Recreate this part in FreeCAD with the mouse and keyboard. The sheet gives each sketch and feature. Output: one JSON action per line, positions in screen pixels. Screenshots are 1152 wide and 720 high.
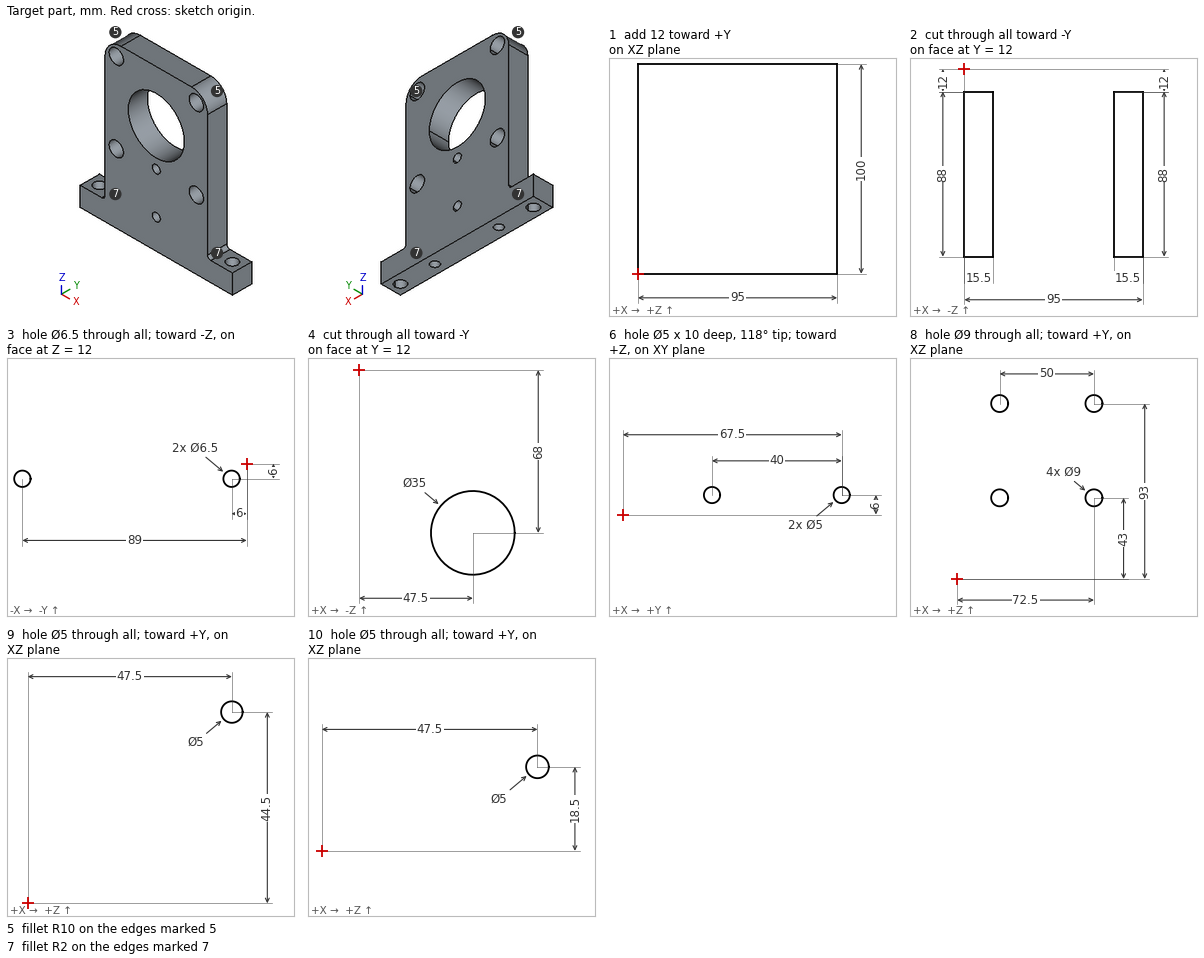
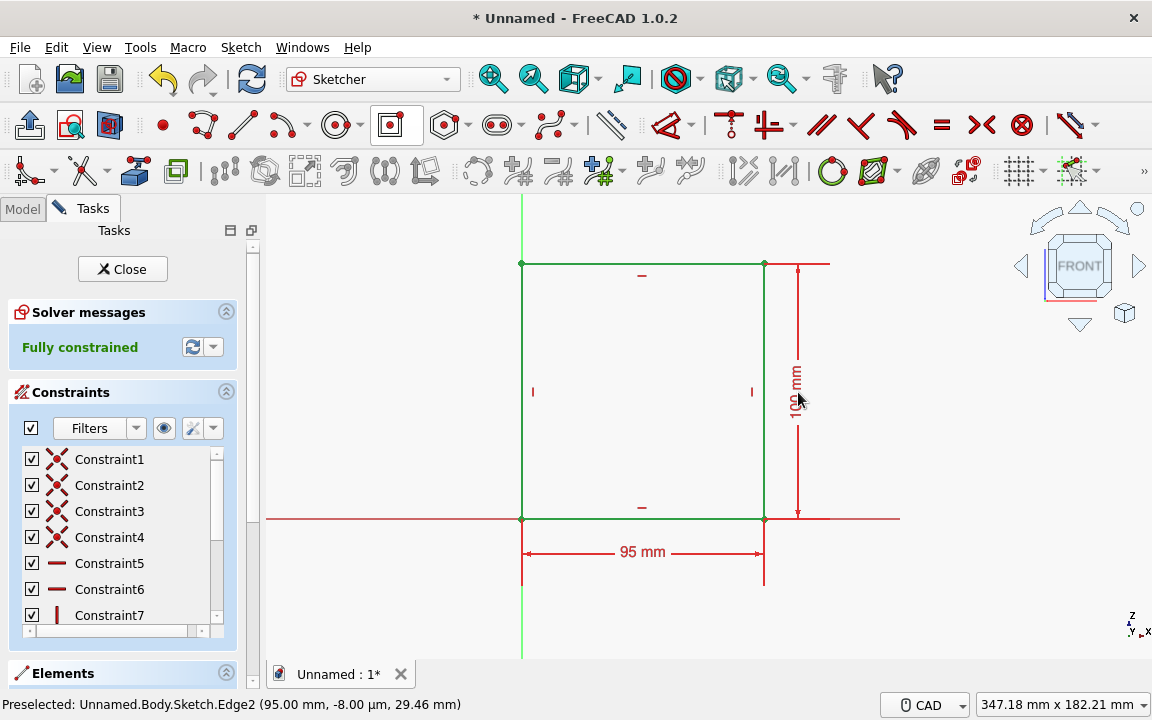
{"action": "left_click", "coordinate": [123, 269]}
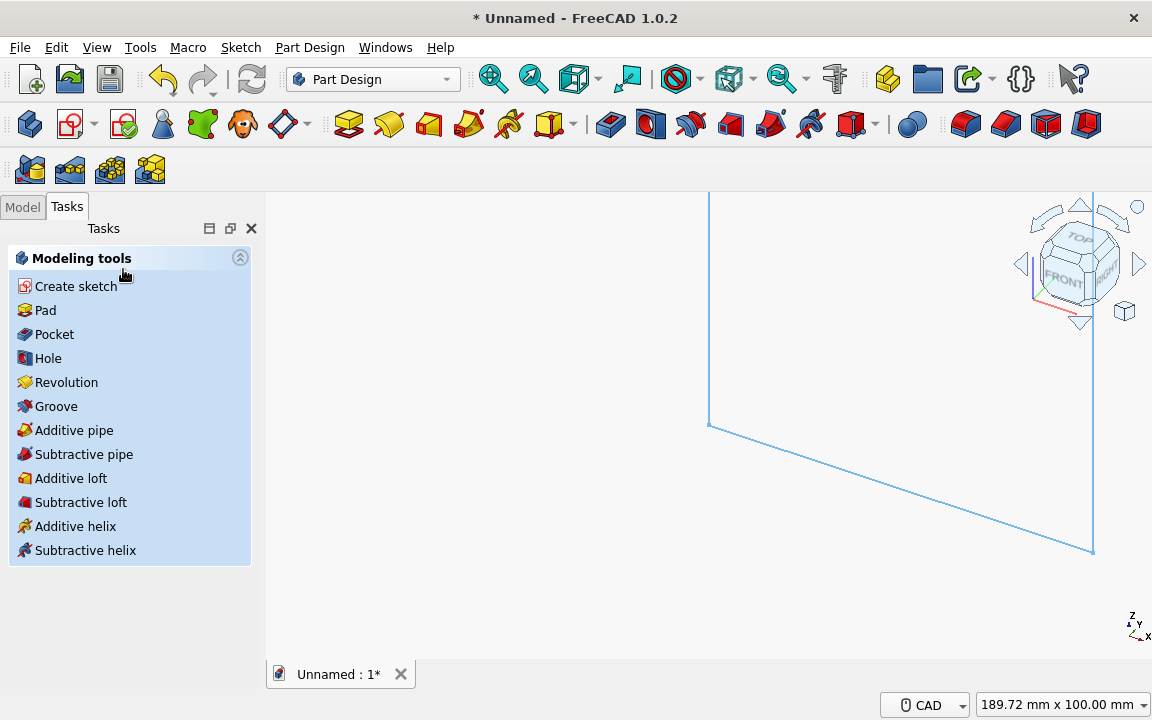
{"action": "left_click", "coordinate": [350, 124]}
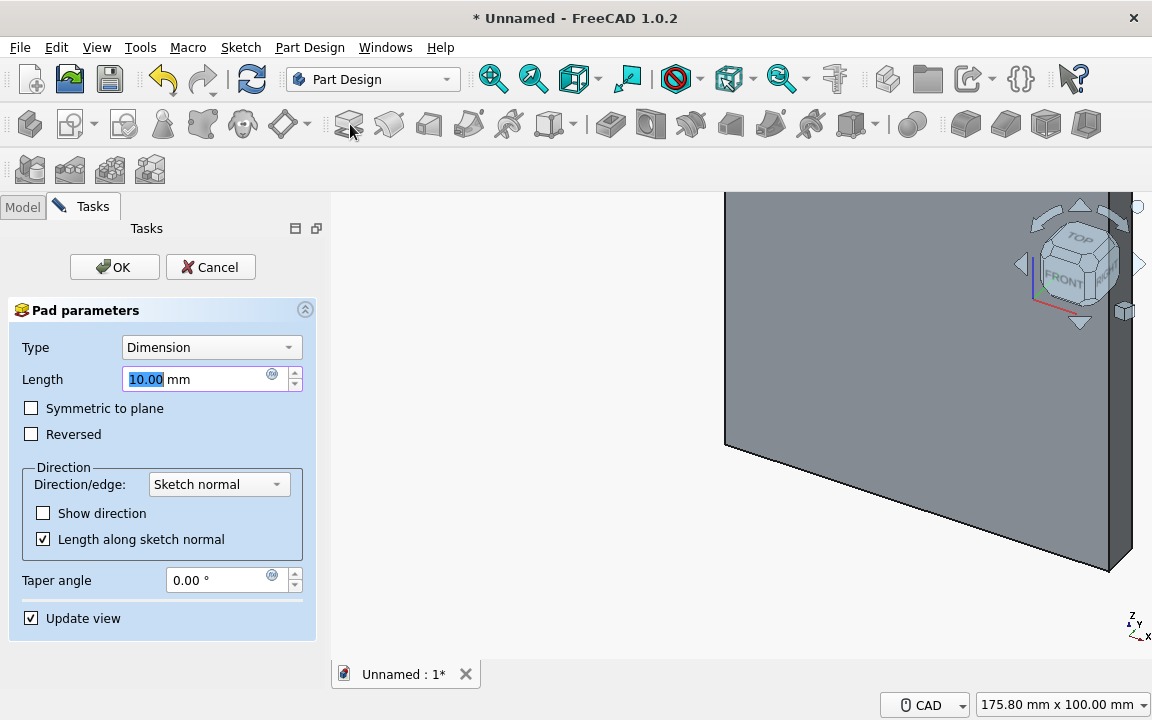
{"action": "type", "text": "12"}
{"action": "key", "text": "Tab"}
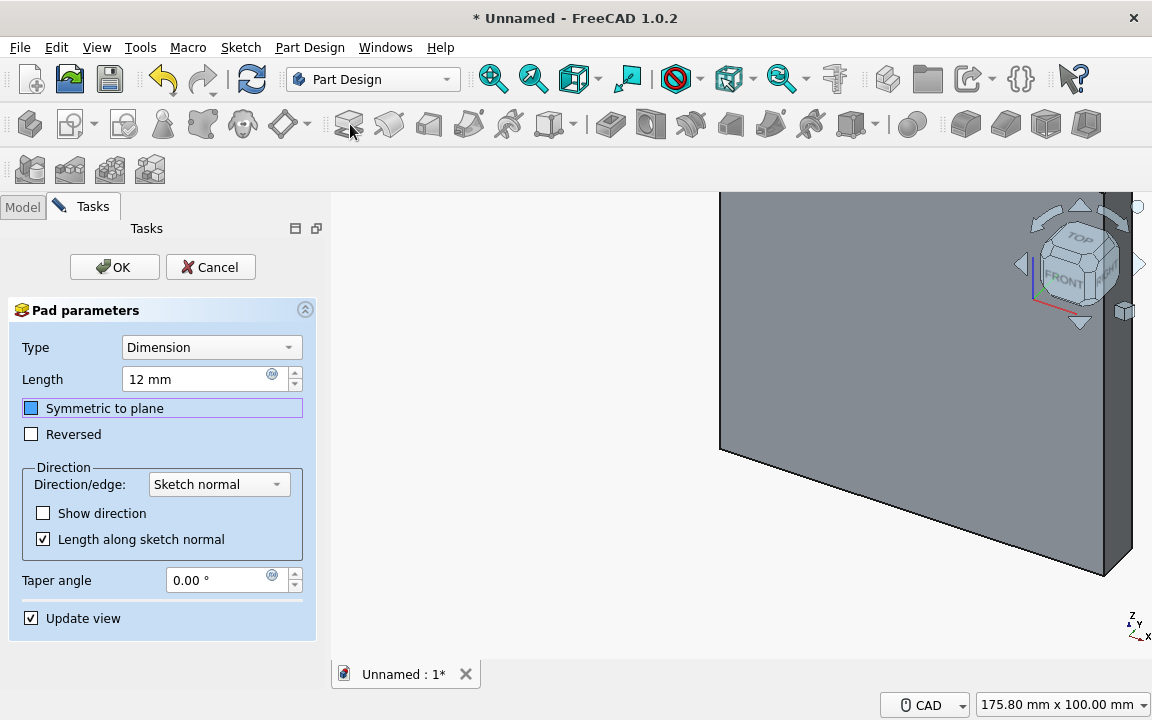
{"action": "left_click", "coordinate": [30, 434]}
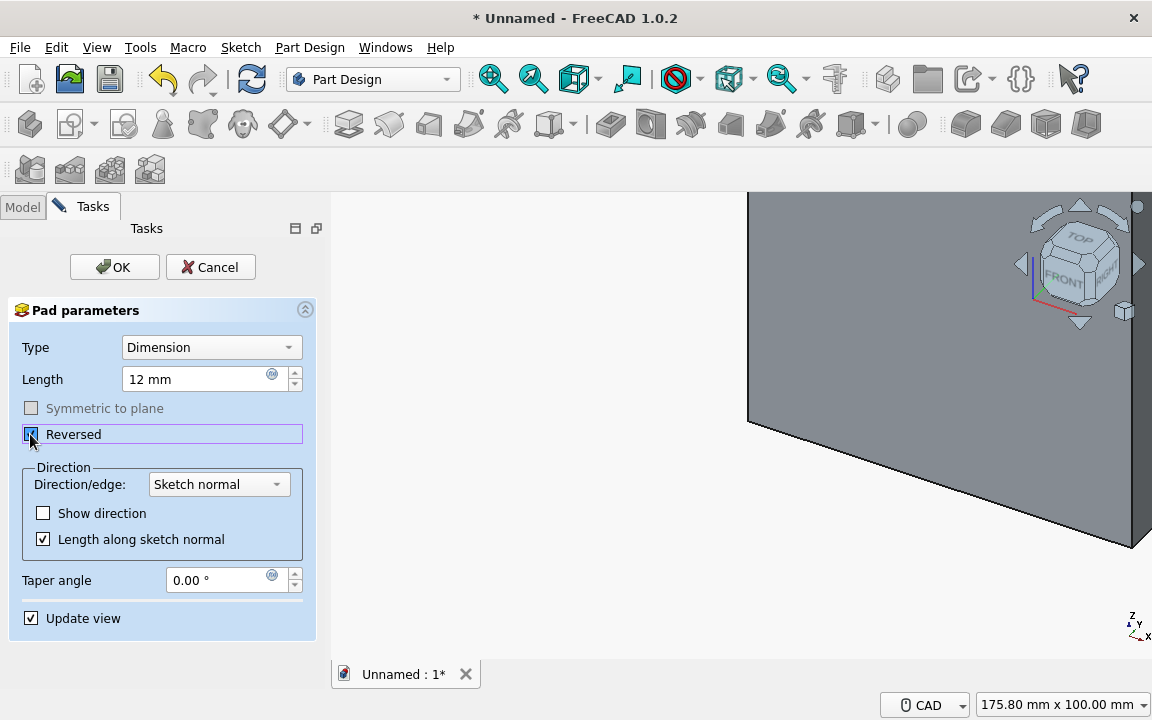
{"action": "left_click", "coordinate": [115, 267]}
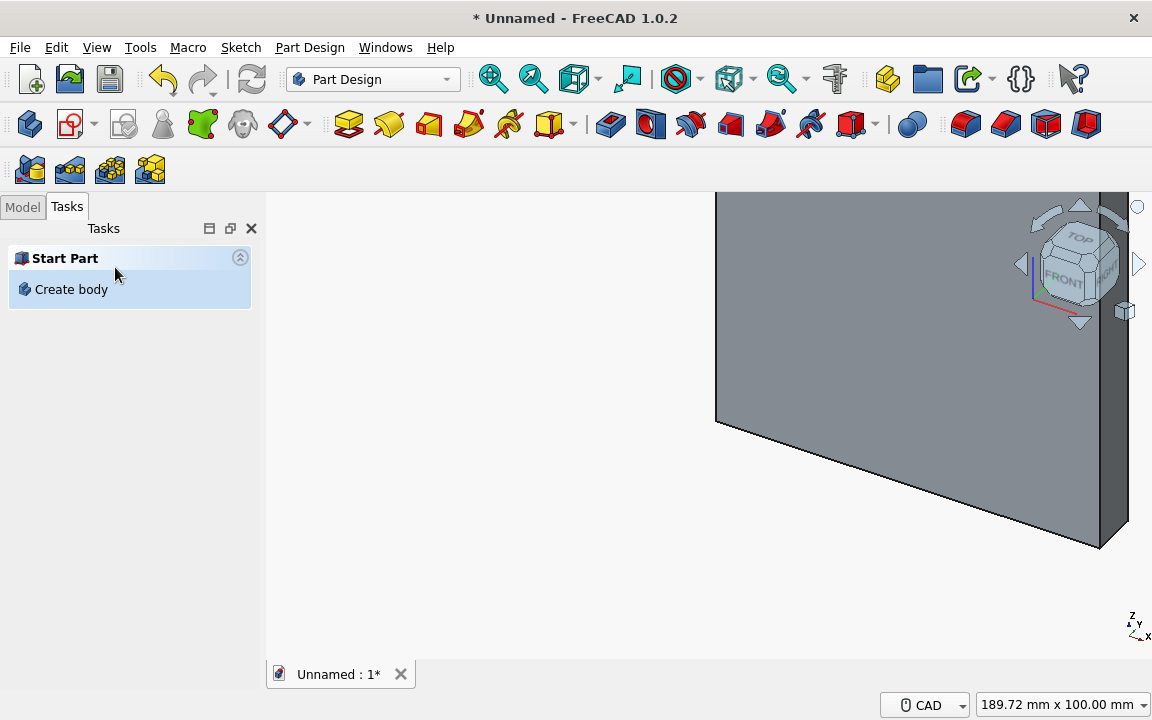
{"action": "left_click", "coordinate": [494, 80]}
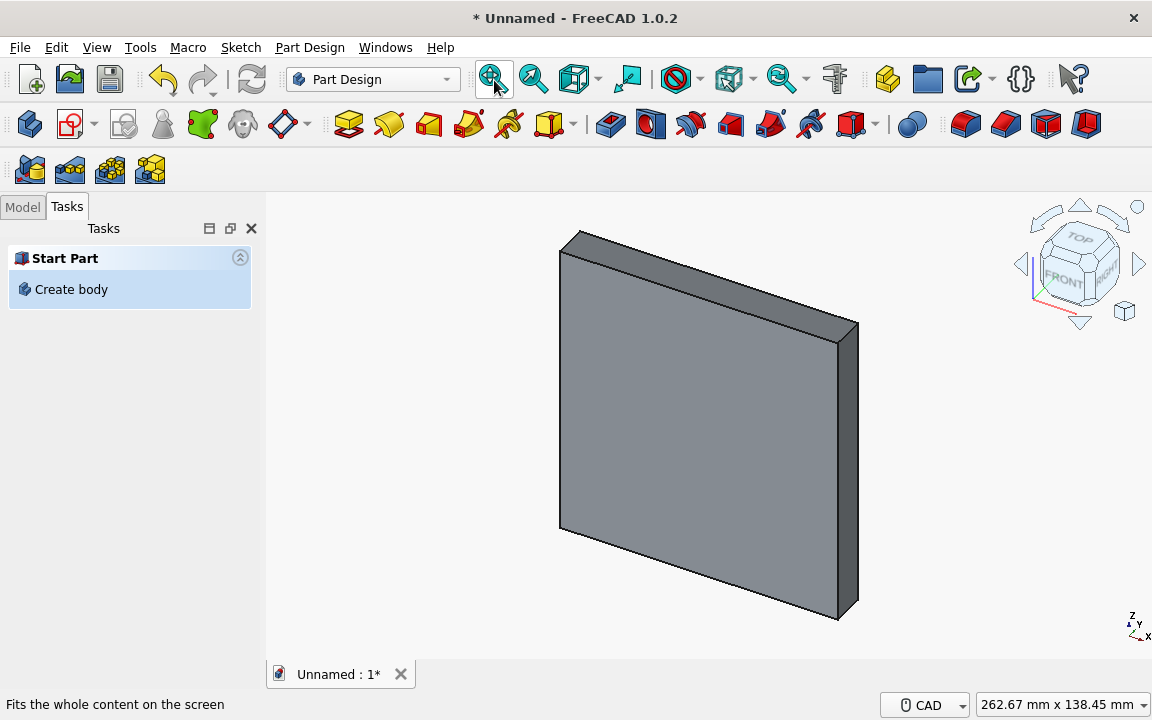
{"action": "key", "text": "4"}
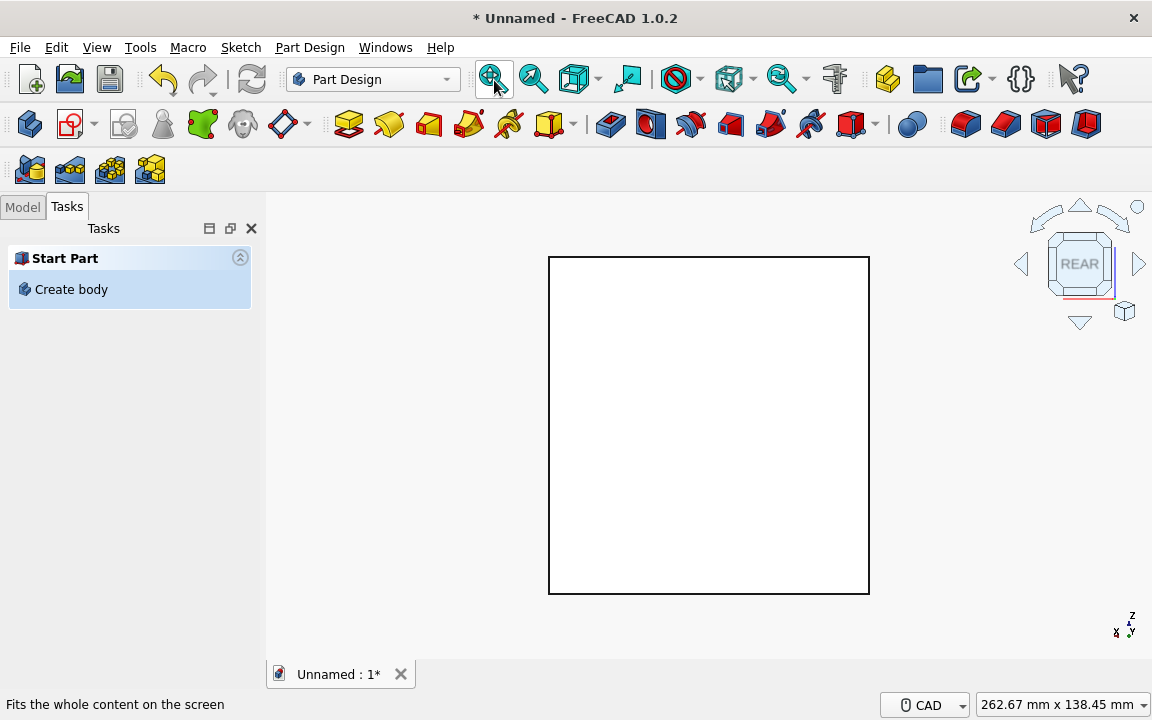
{"action": "left_click", "coordinate": [709, 425]}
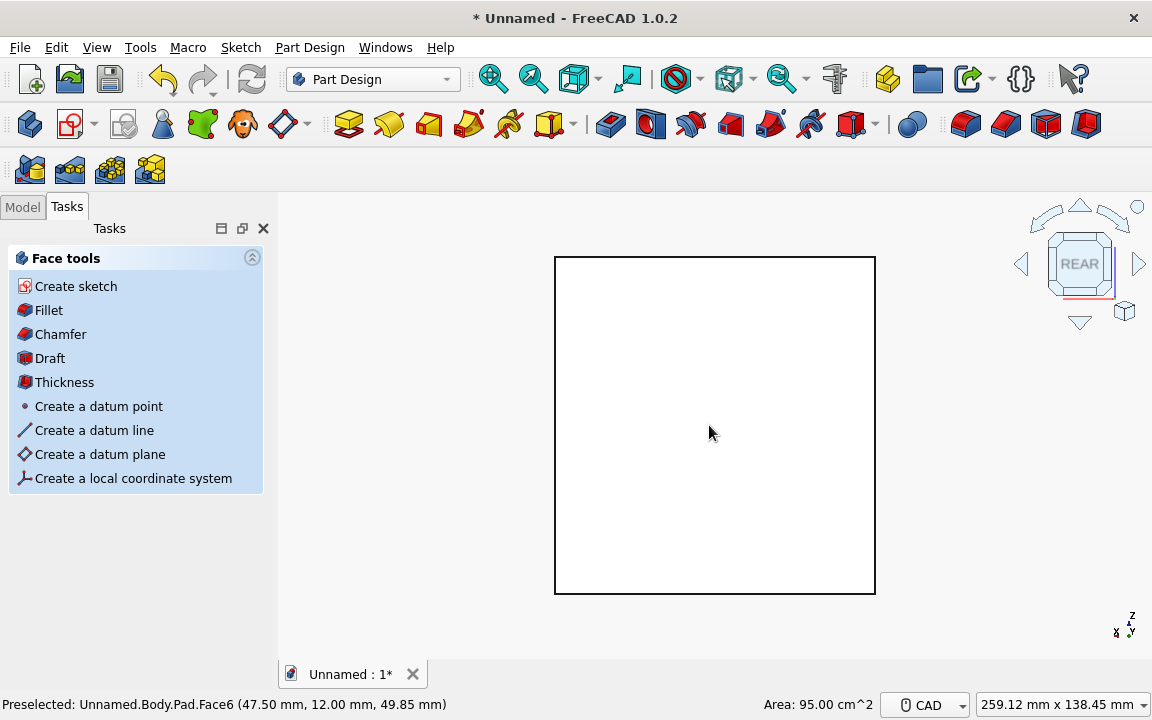
{"action": "left_click", "coordinate": [70, 124]}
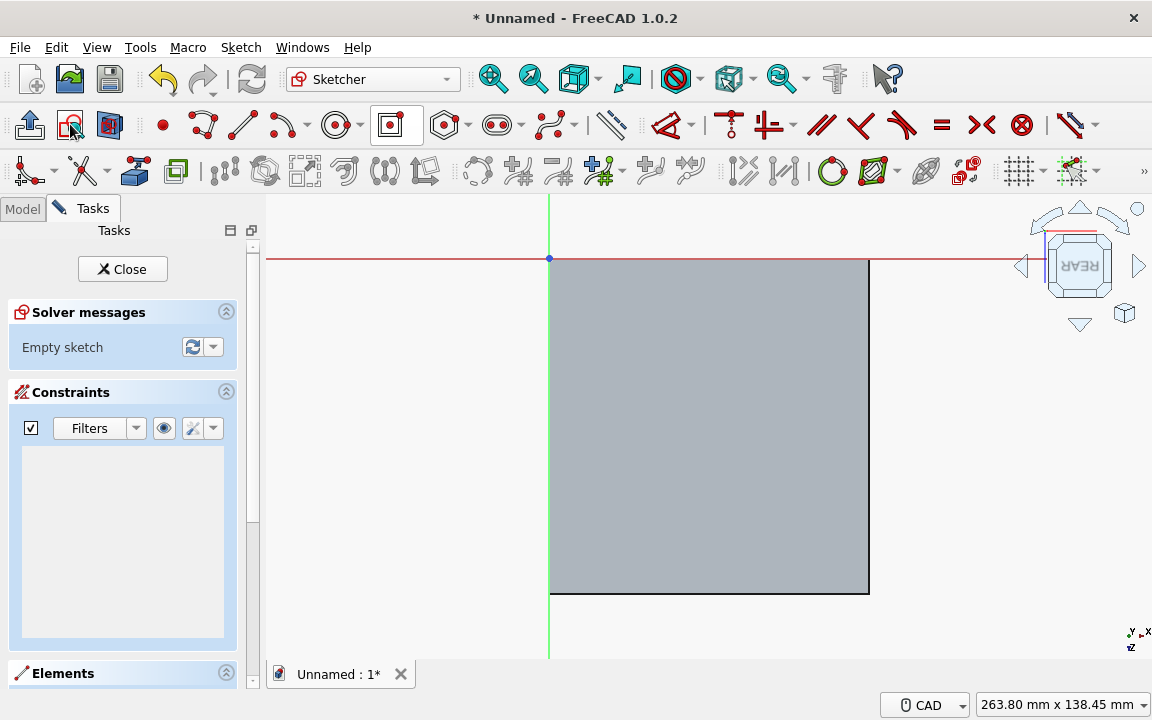
{"action": "key", "text": "g r"}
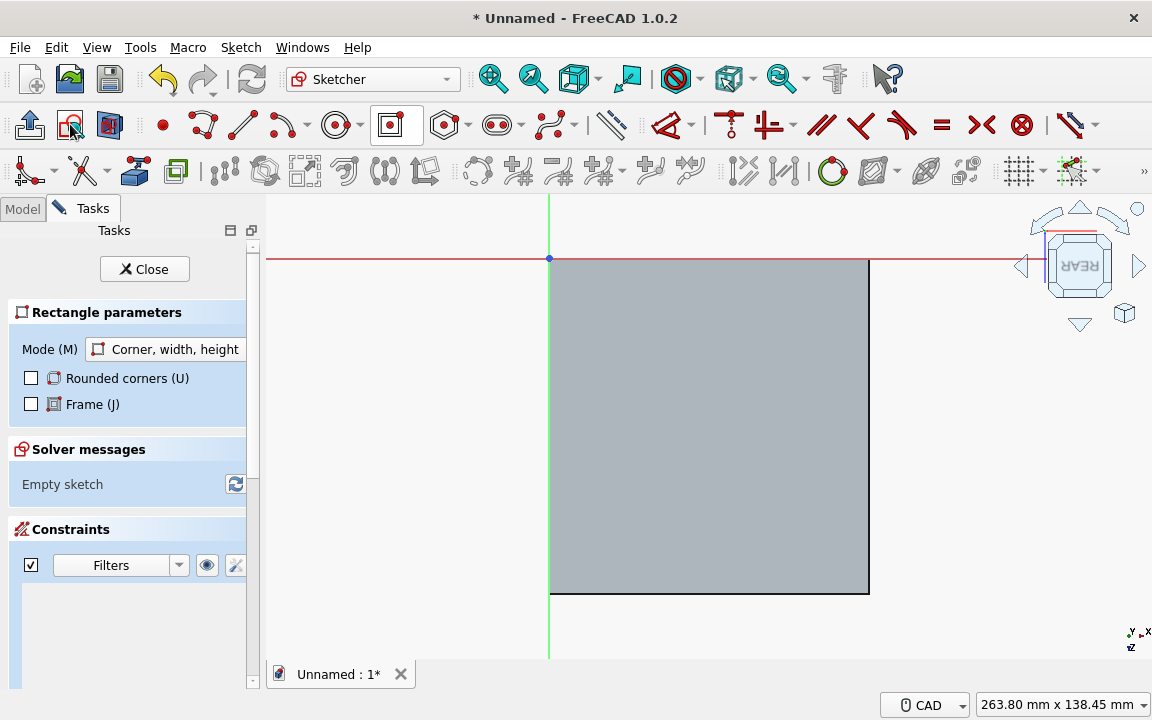
{"action": "left_click", "coordinate": [549, 299]}
{"action": "left_click", "coordinate": [602, 594]}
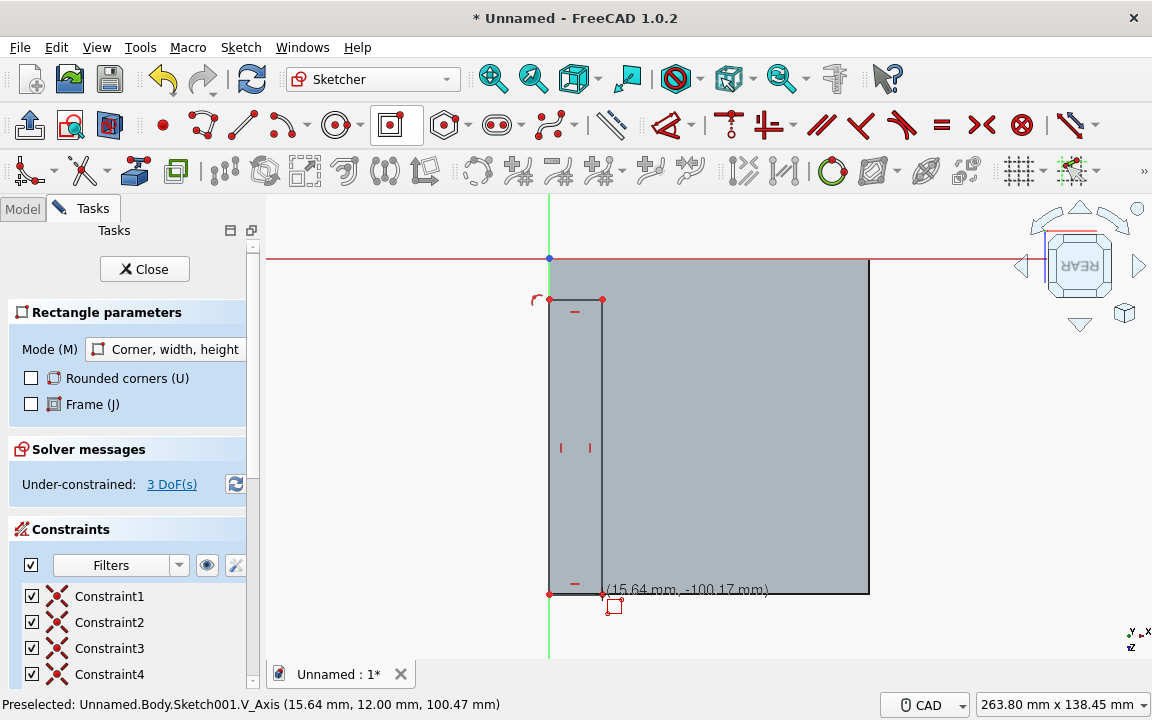
{"action": "left_click", "coordinate": [816, 299]}
{"action": "left_click", "coordinate": [869, 594]}
{"action": "key", "text": "Escape"}